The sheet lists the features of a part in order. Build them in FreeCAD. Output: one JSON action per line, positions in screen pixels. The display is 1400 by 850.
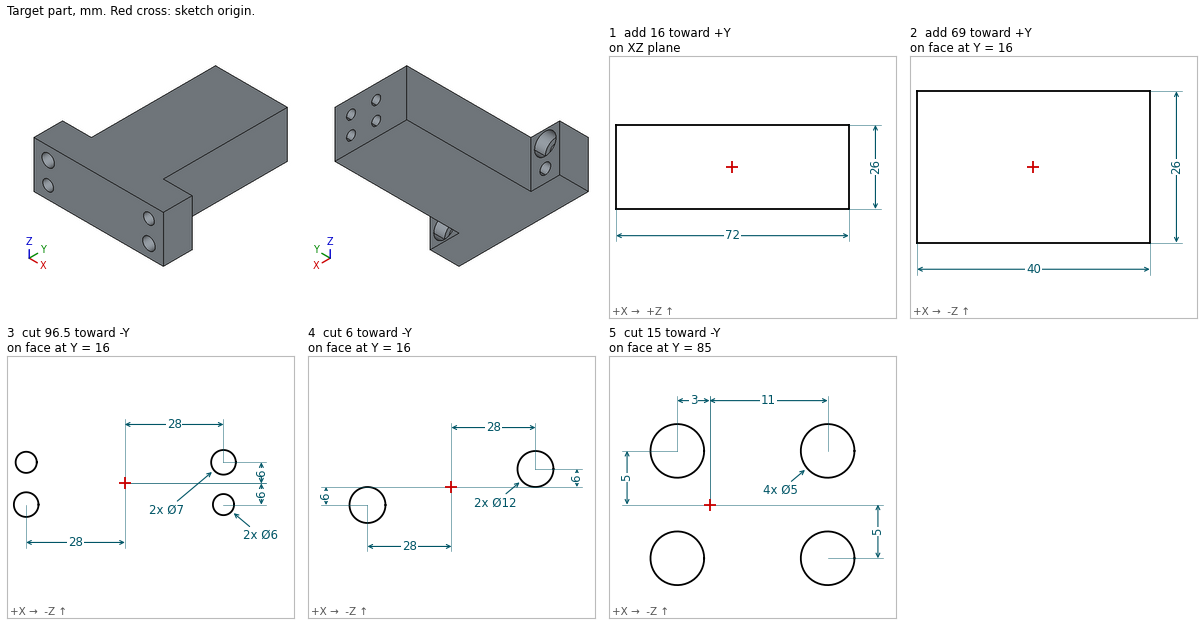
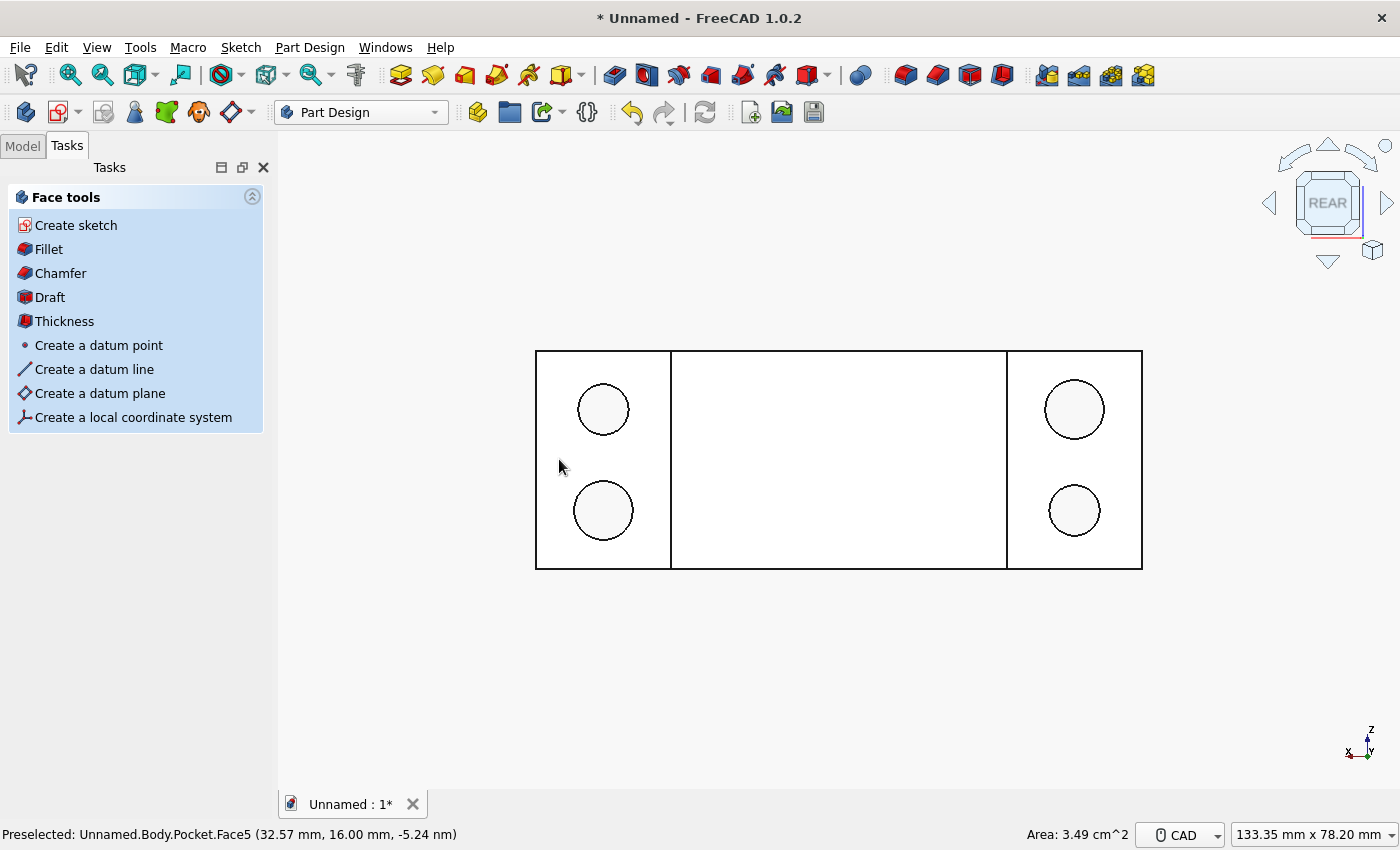
{"action": "left_click", "coordinate": [58, 112]}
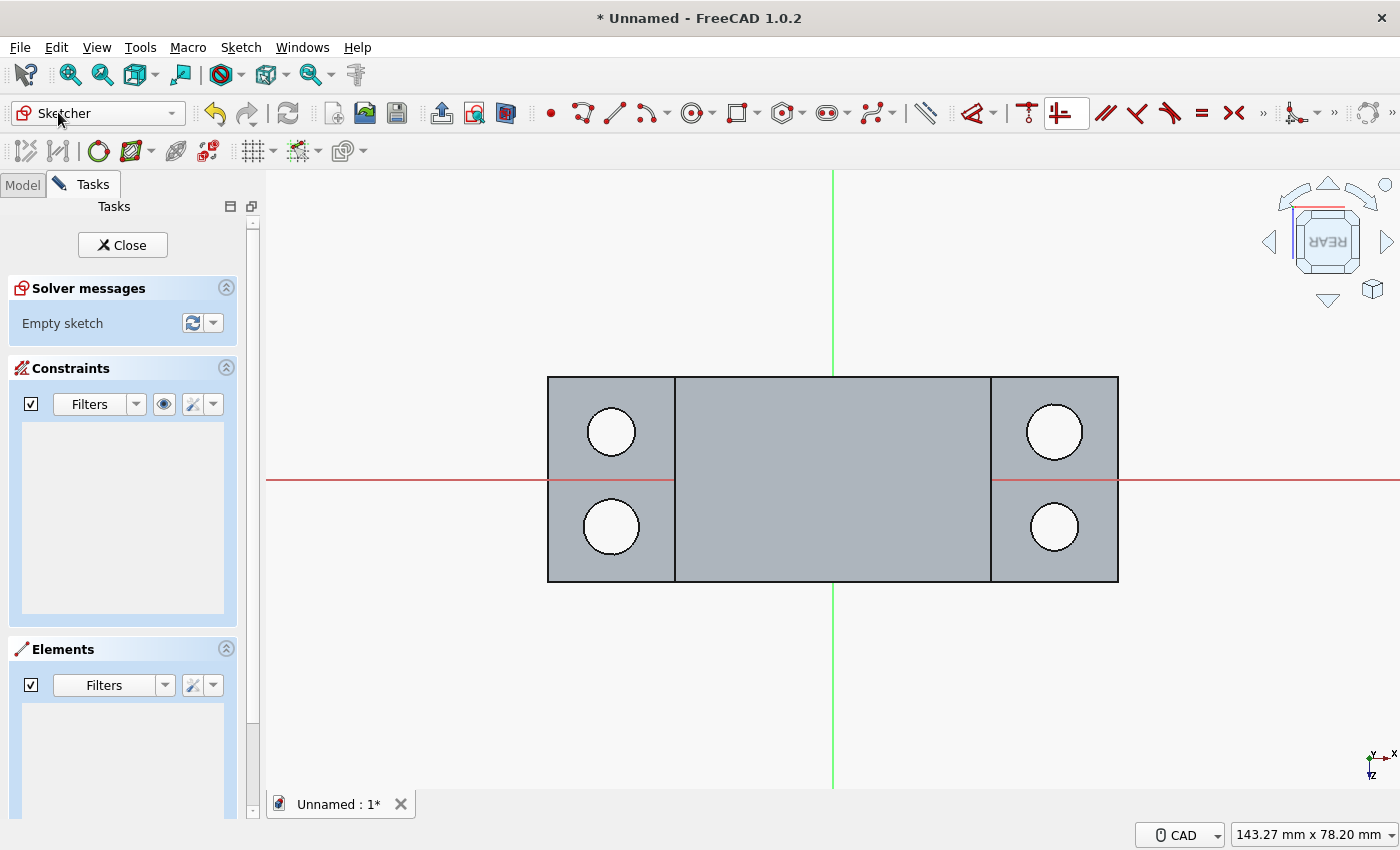
{"action": "left_click", "coordinate": [506, 114]}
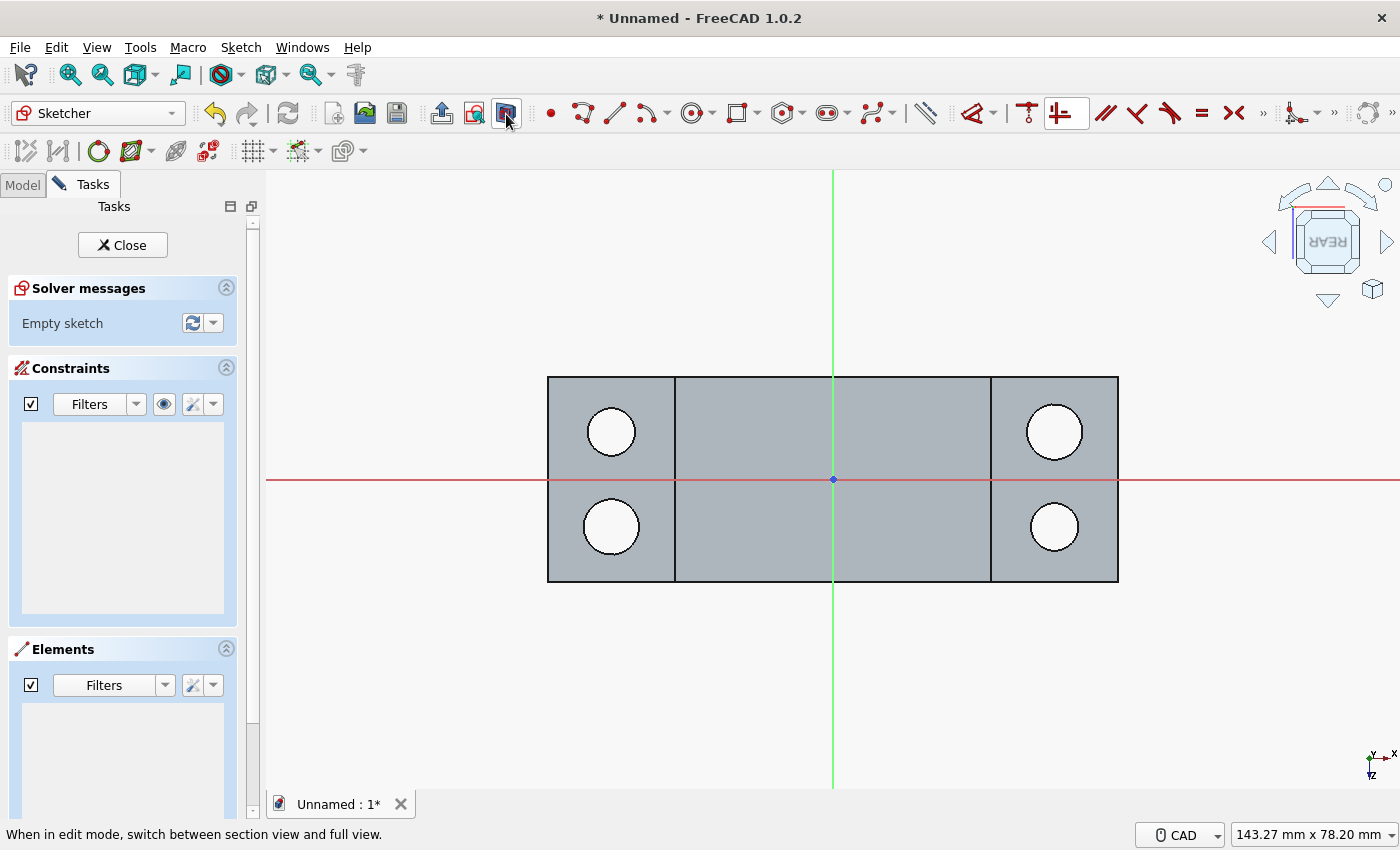
{"action": "left_click", "coordinate": [692, 114]}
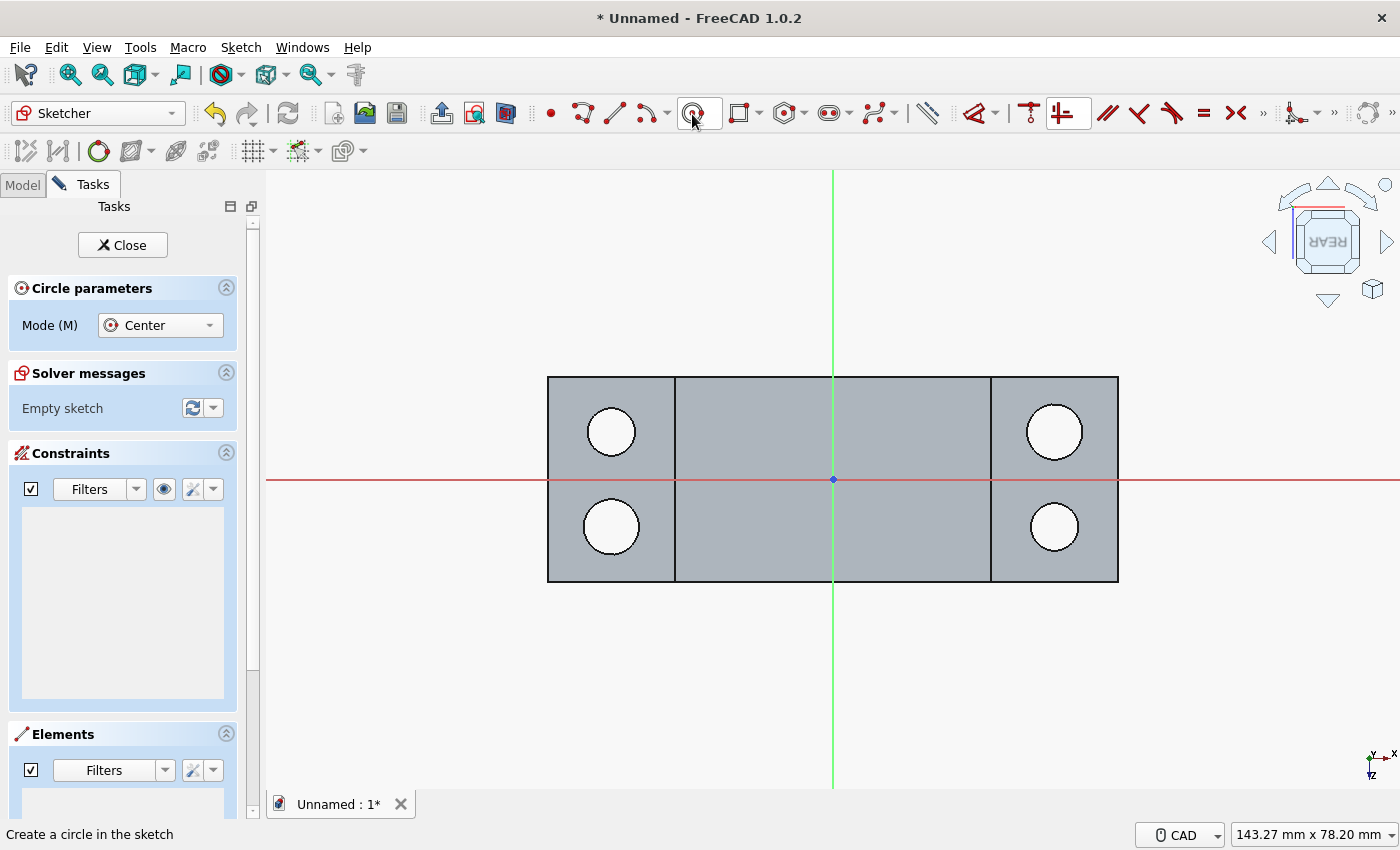
{"action": "left_click", "coordinate": [1055, 432]}
{"action": "mouse_move", "coordinate": [1088, 398]}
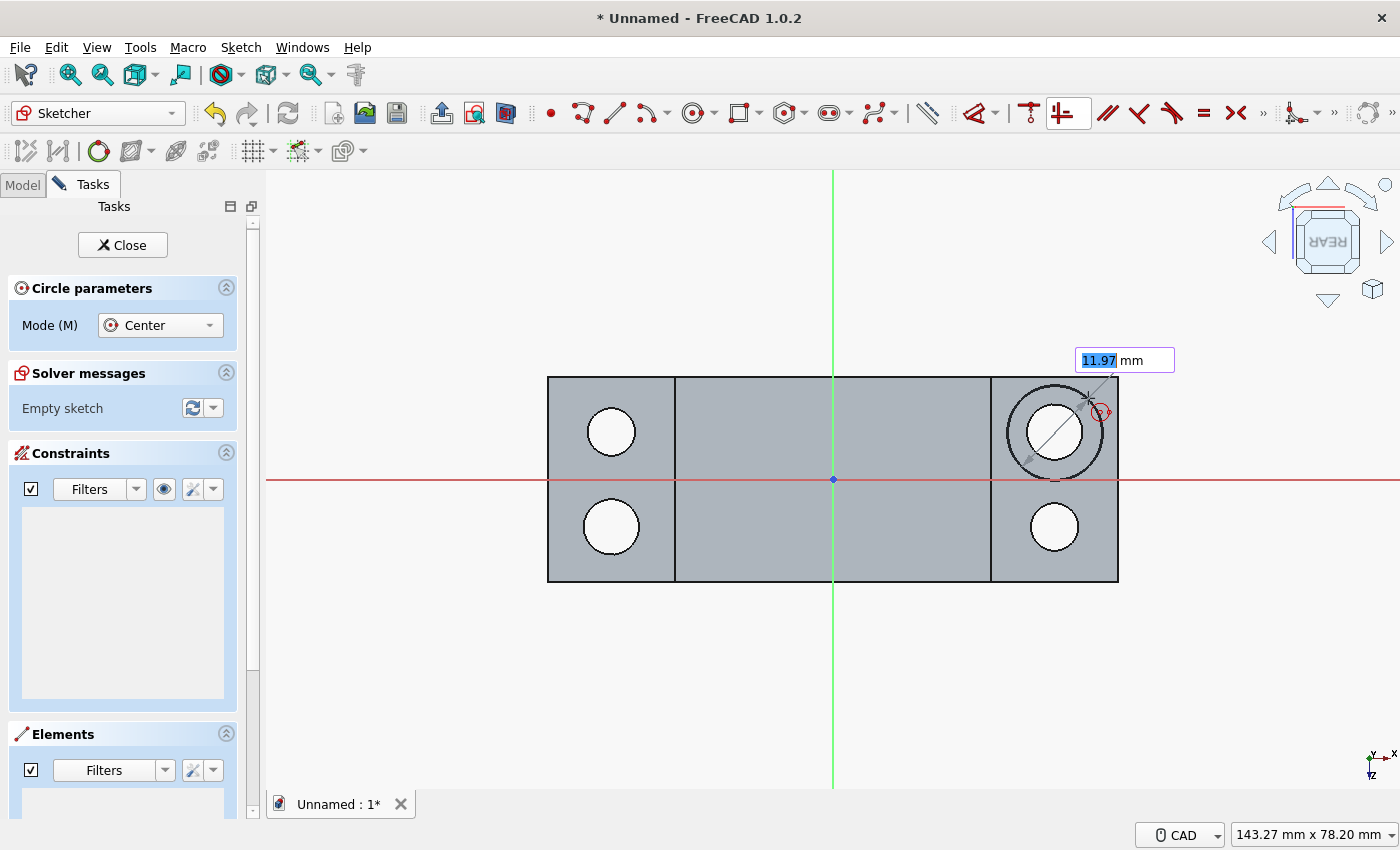
{"action": "type", "text": "12"}
{"action": "key", "text": "Return"}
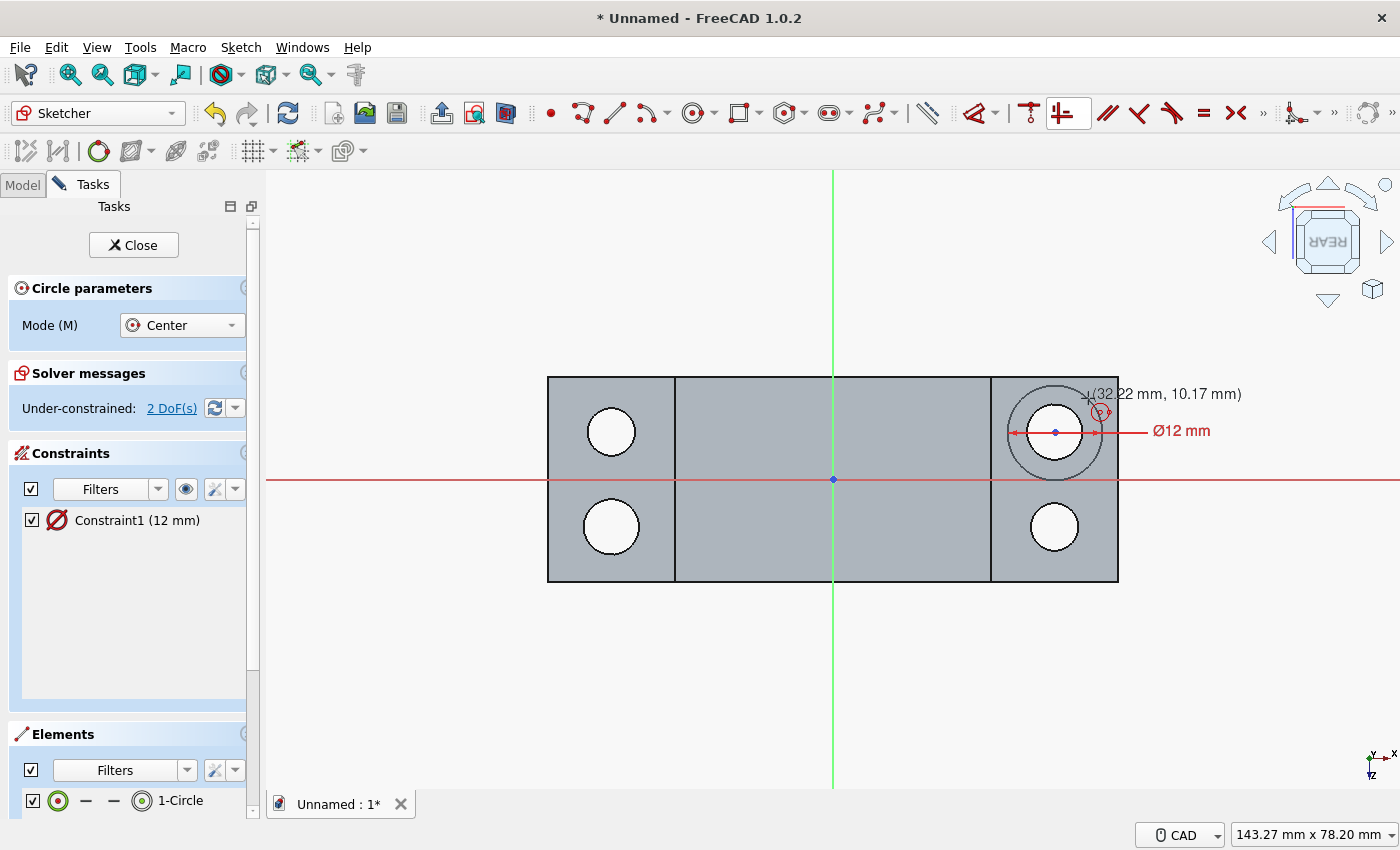
{"action": "left_click", "coordinate": [611, 527]}
{"action": "mouse_move", "coordinate": [645, 561]}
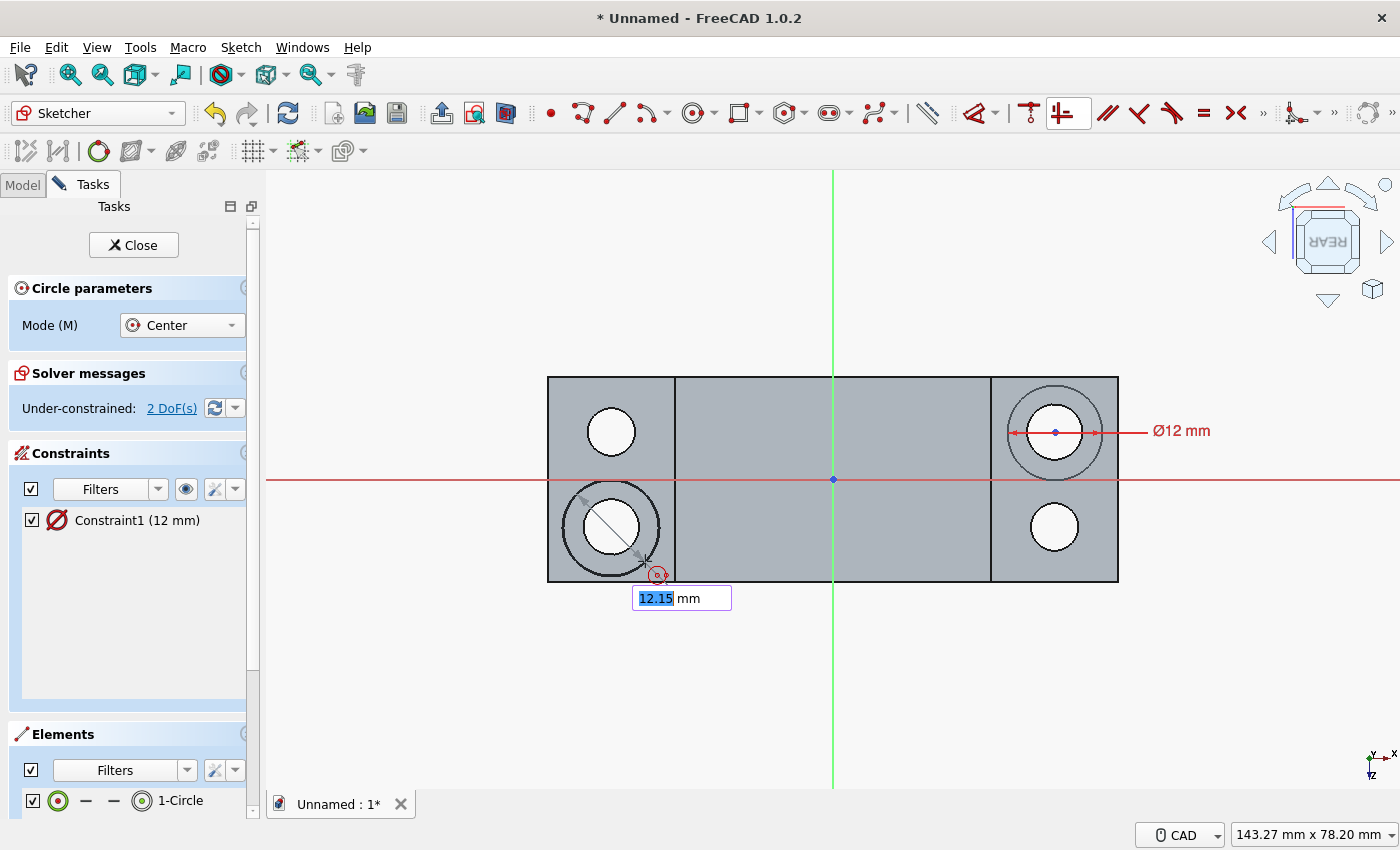
{"action": "type", "text": "12"}
{"action": "key", "text": "Return"}
{"action": "key", "text": "Escape"}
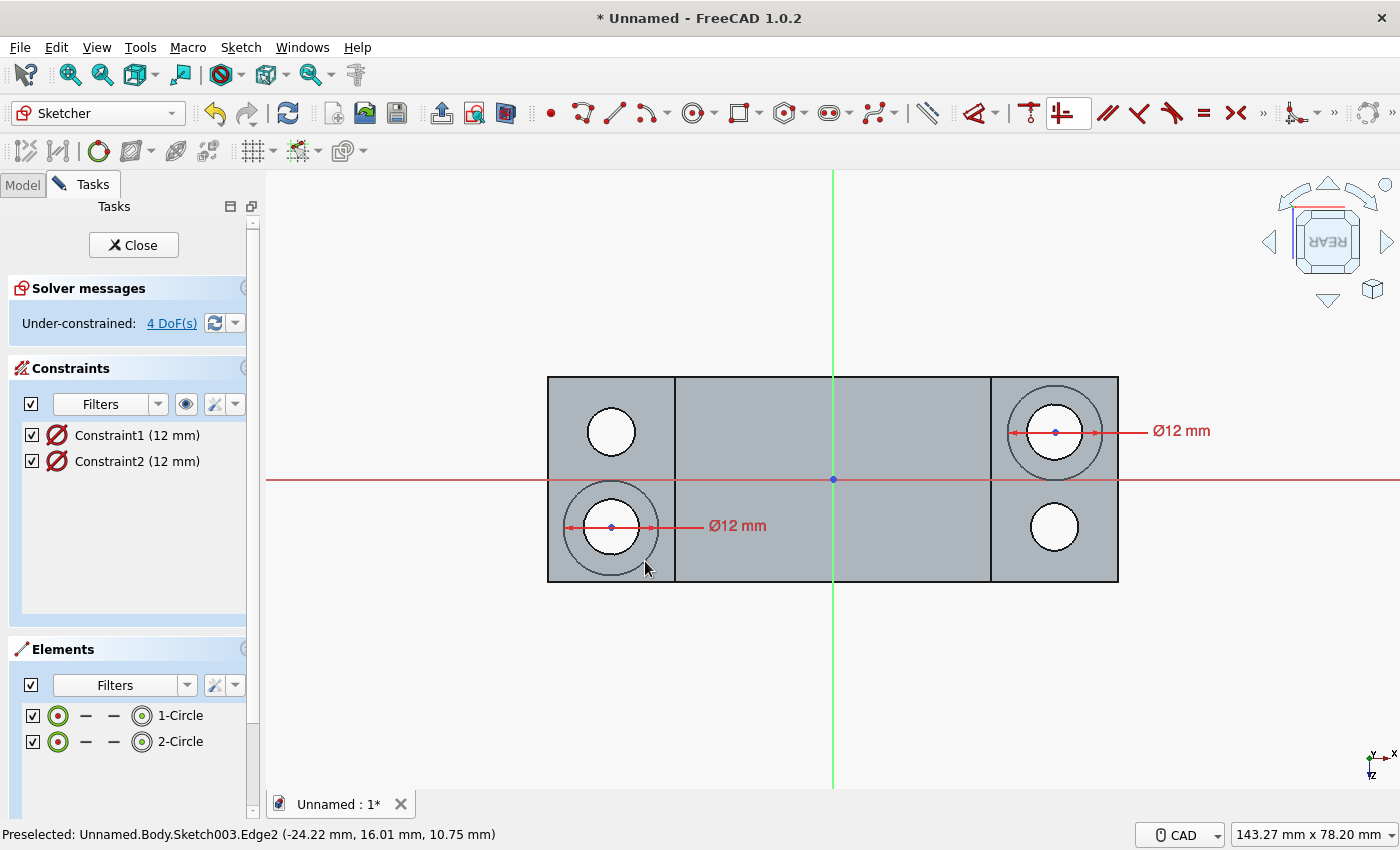
{"action": "key", "text": "d"}